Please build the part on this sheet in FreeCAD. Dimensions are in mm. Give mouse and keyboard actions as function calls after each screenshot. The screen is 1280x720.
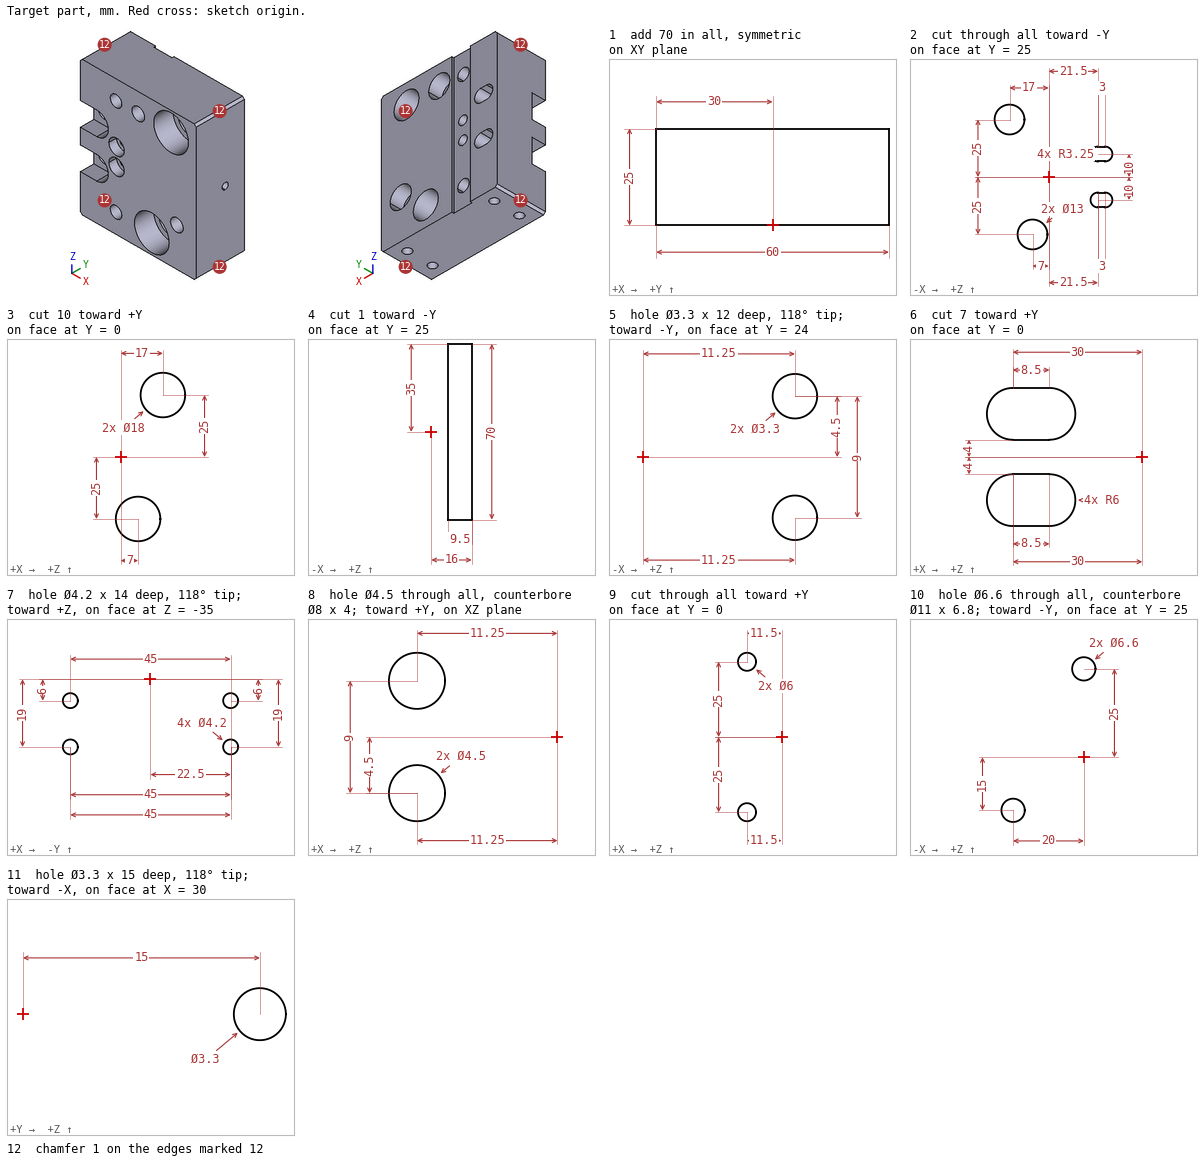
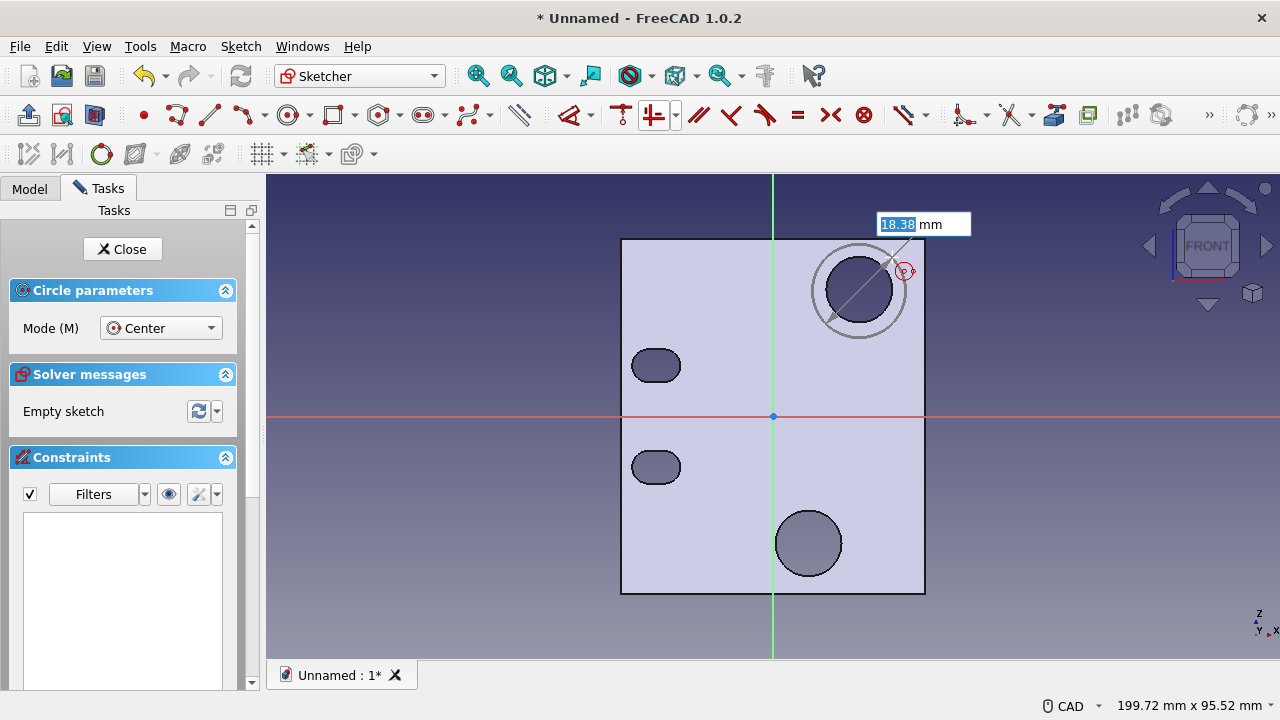
text(18)
key(Return)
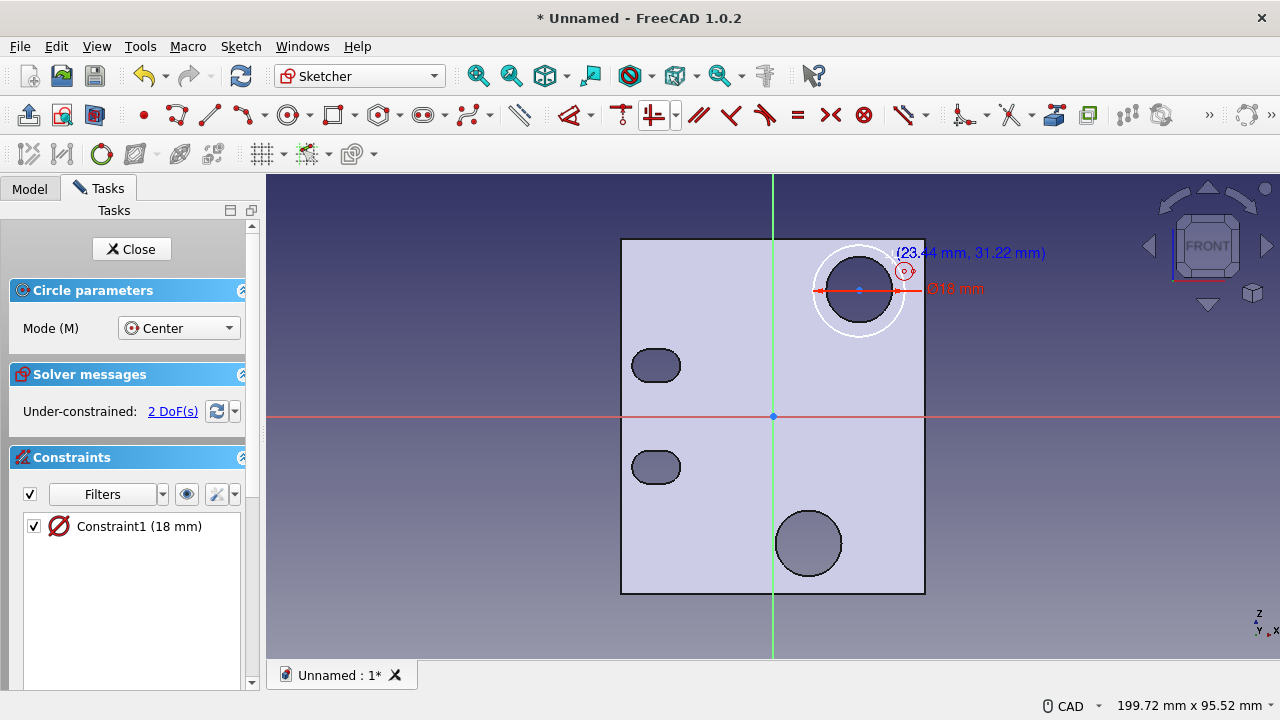
click(809, 543)
move(841, 511)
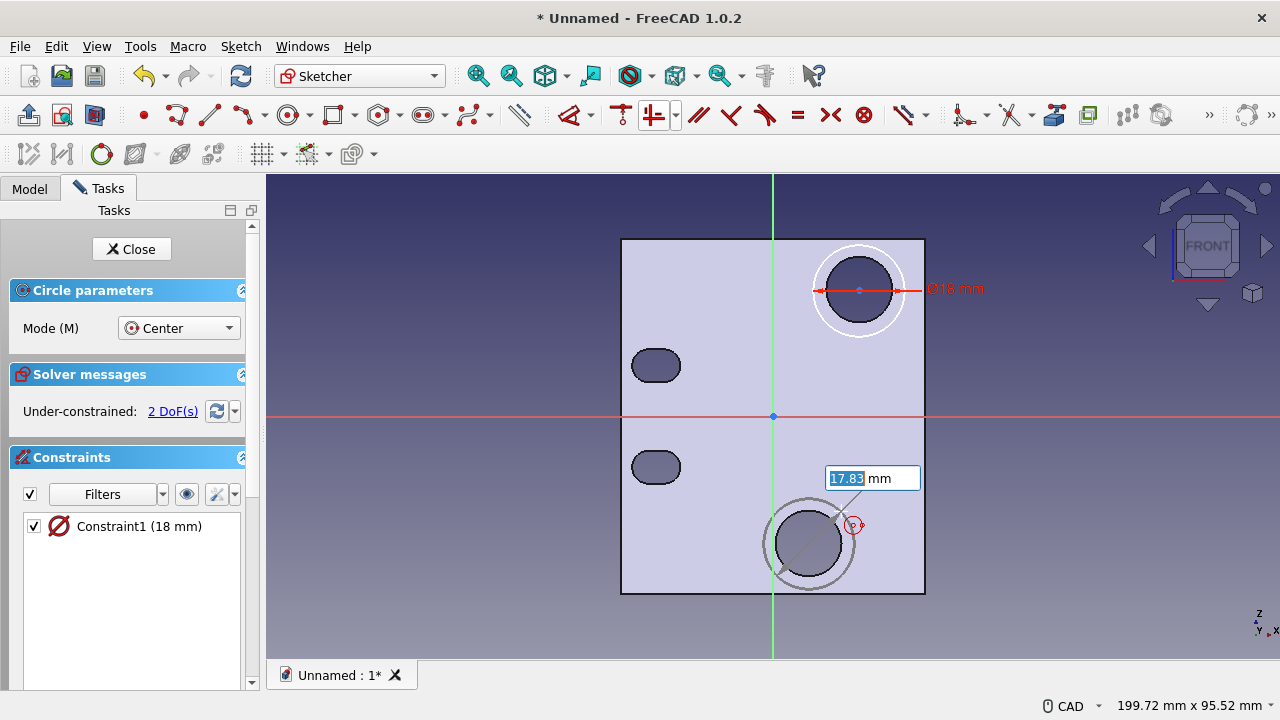
text(18)
key(Return)
key(Escape)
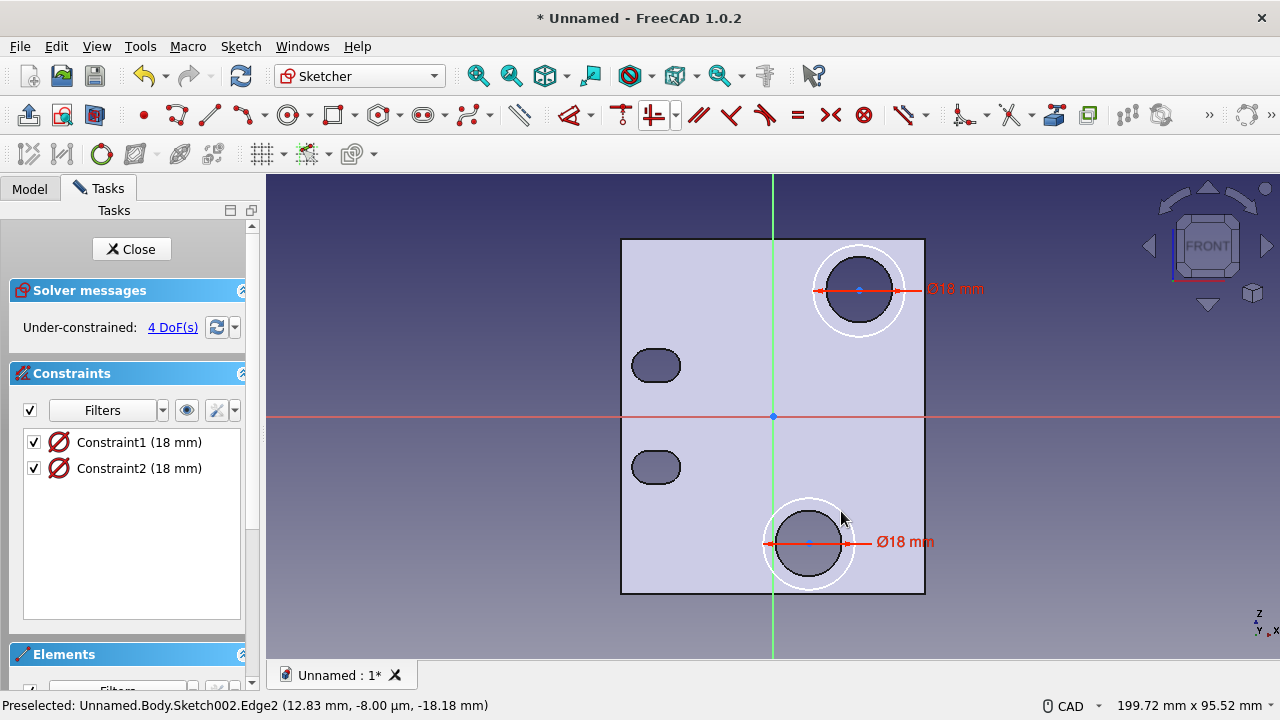
key(d)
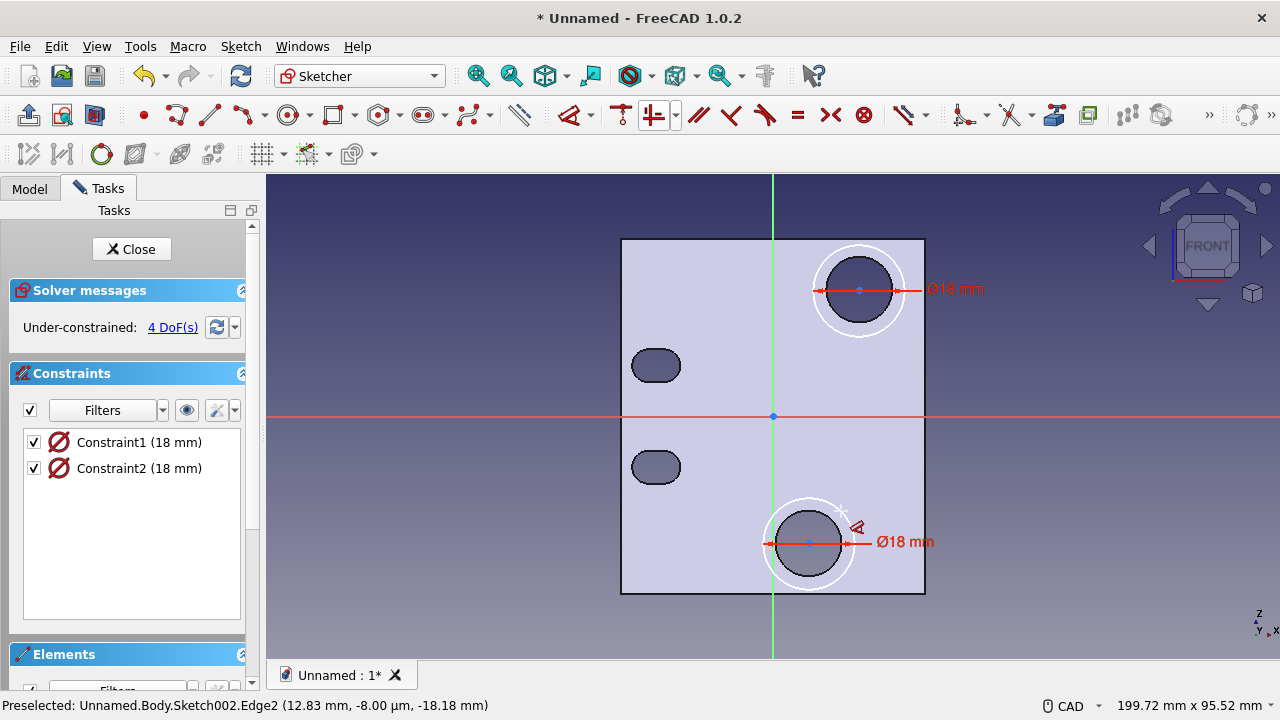
click(809, 544)
click(791, 382)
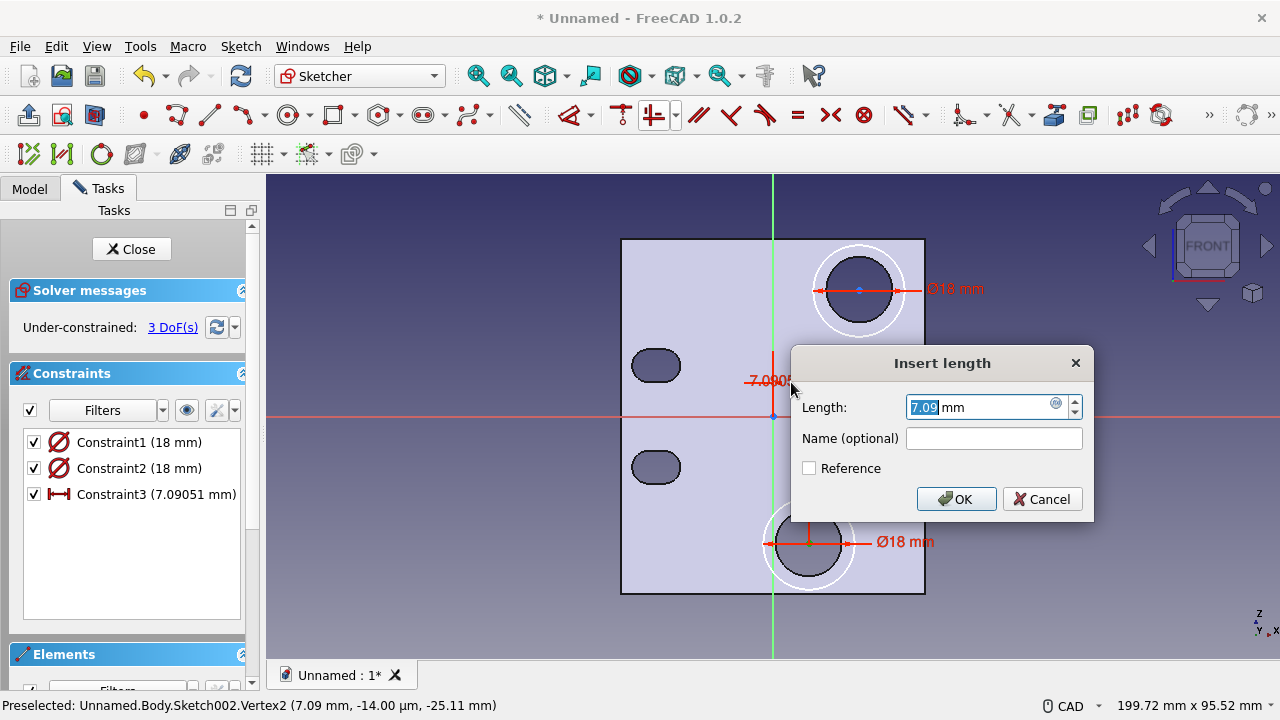
text(7)
key(Return)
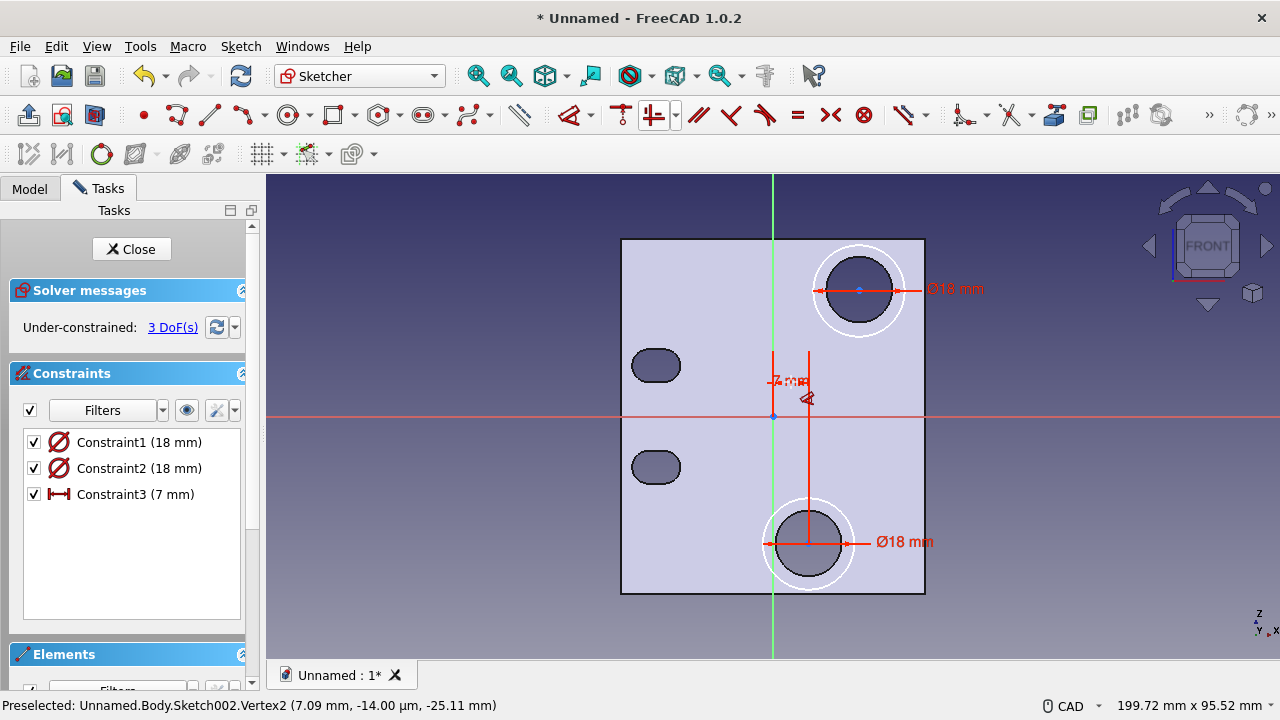
click(859, 291)
click(796, 257)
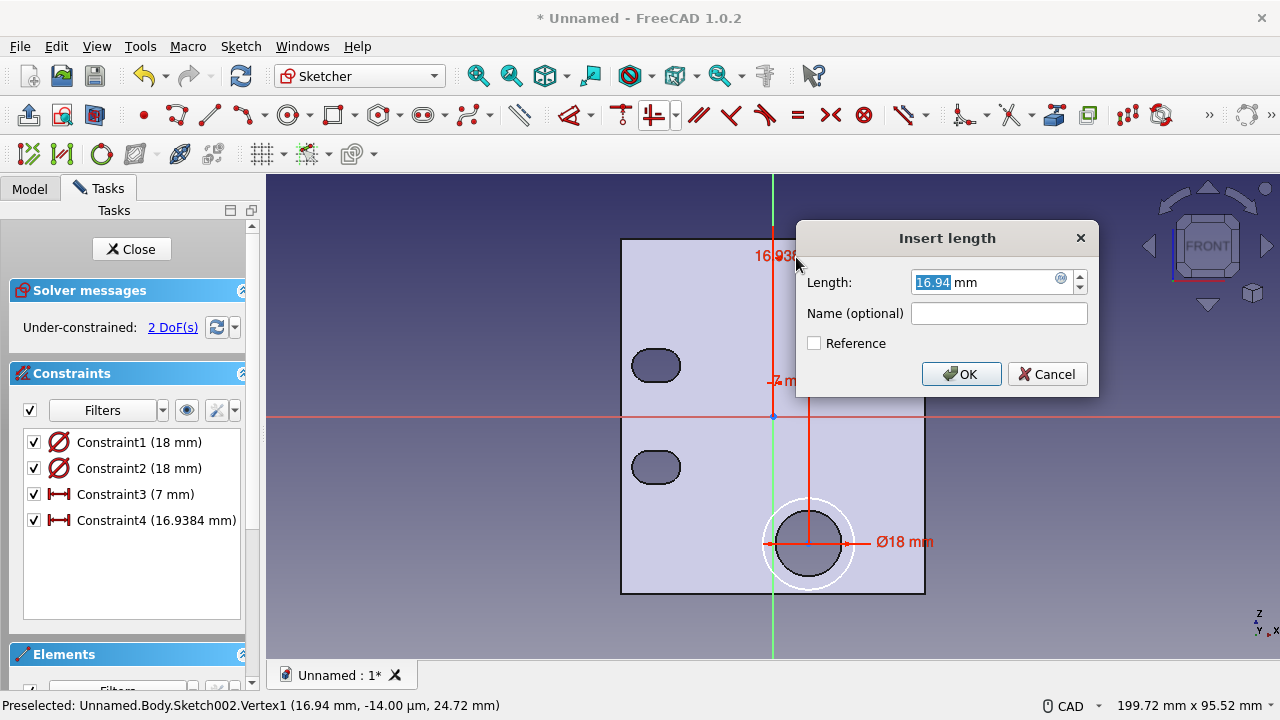
text(17)
key(Return)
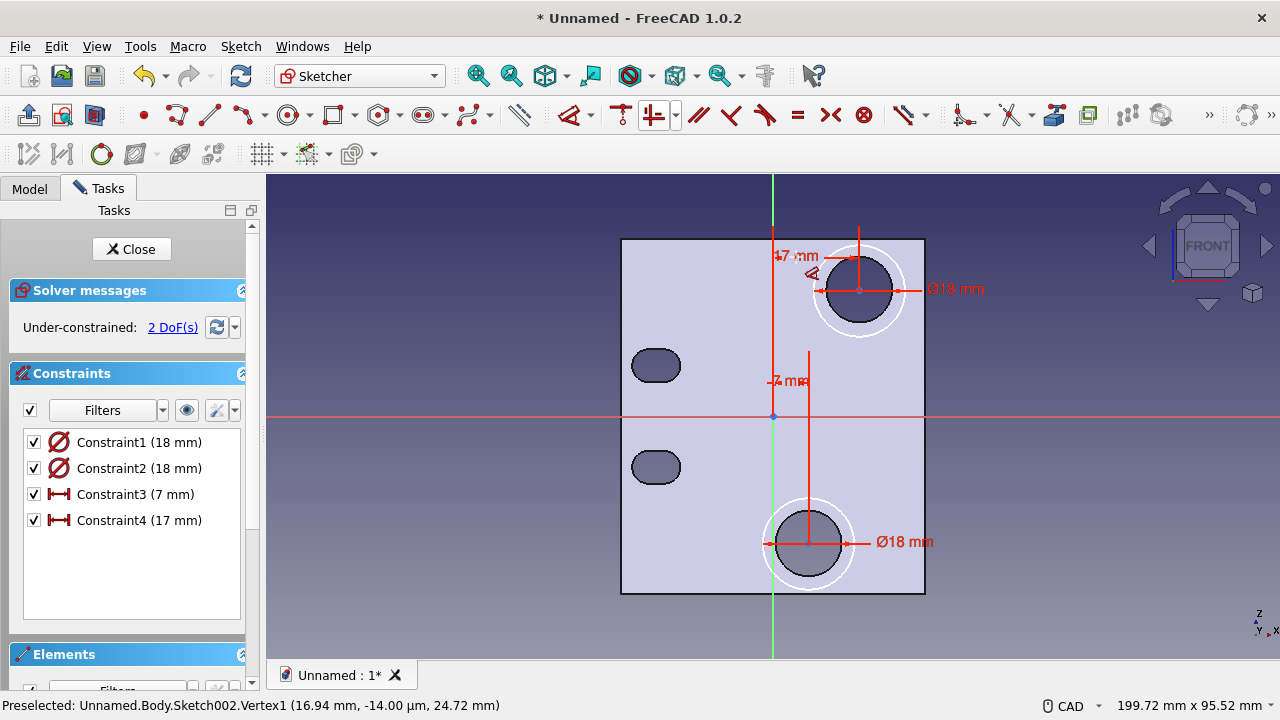
click(859, 291)
click(739, 354)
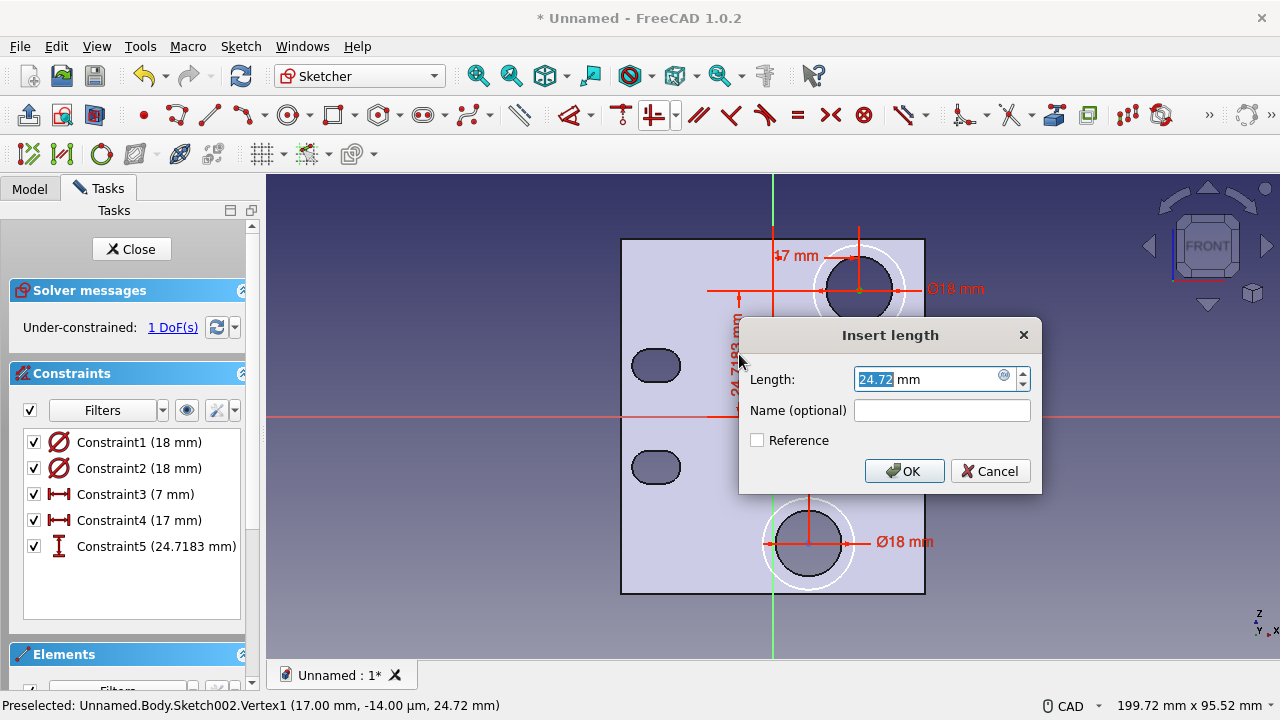
text(25)
key(Return)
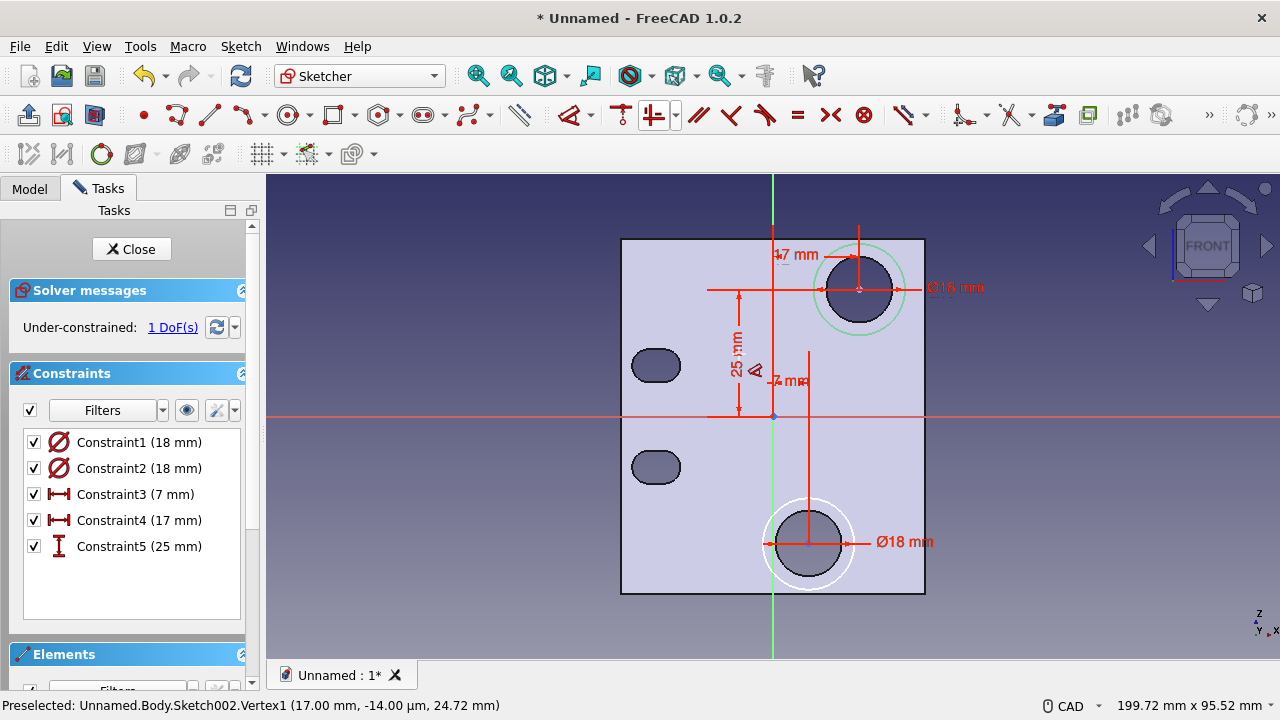
click(809, 544)
click(739, 480)